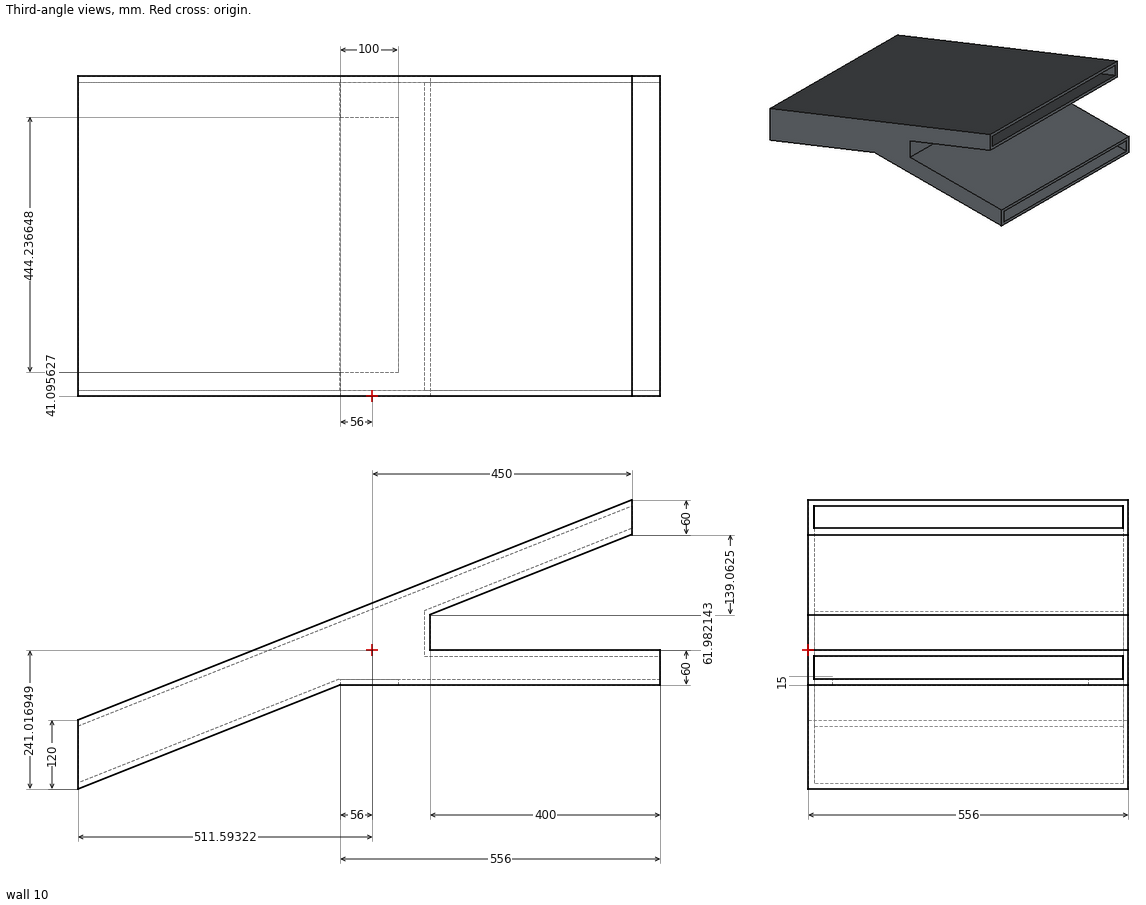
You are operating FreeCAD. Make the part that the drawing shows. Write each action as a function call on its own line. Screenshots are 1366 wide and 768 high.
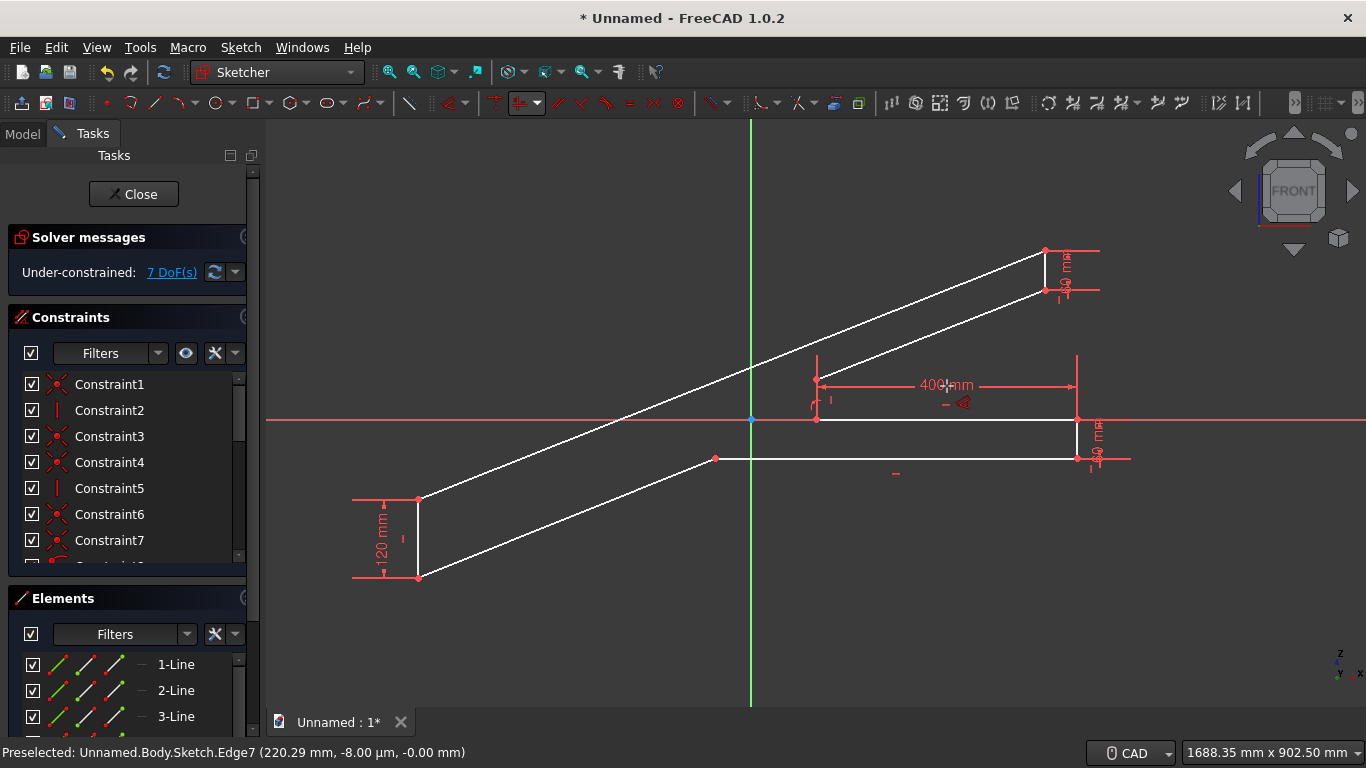
click(969, 459)
click(896, 493)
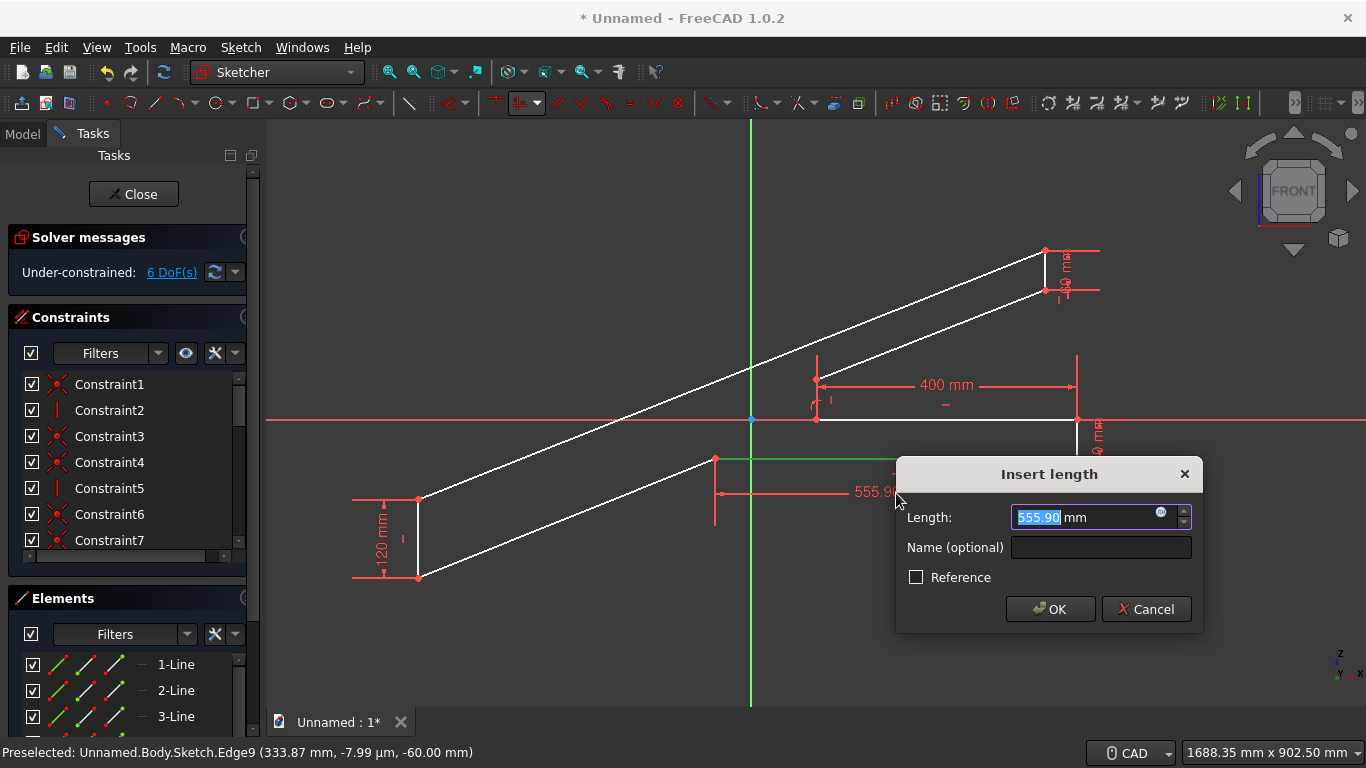
text(556)
key(Return)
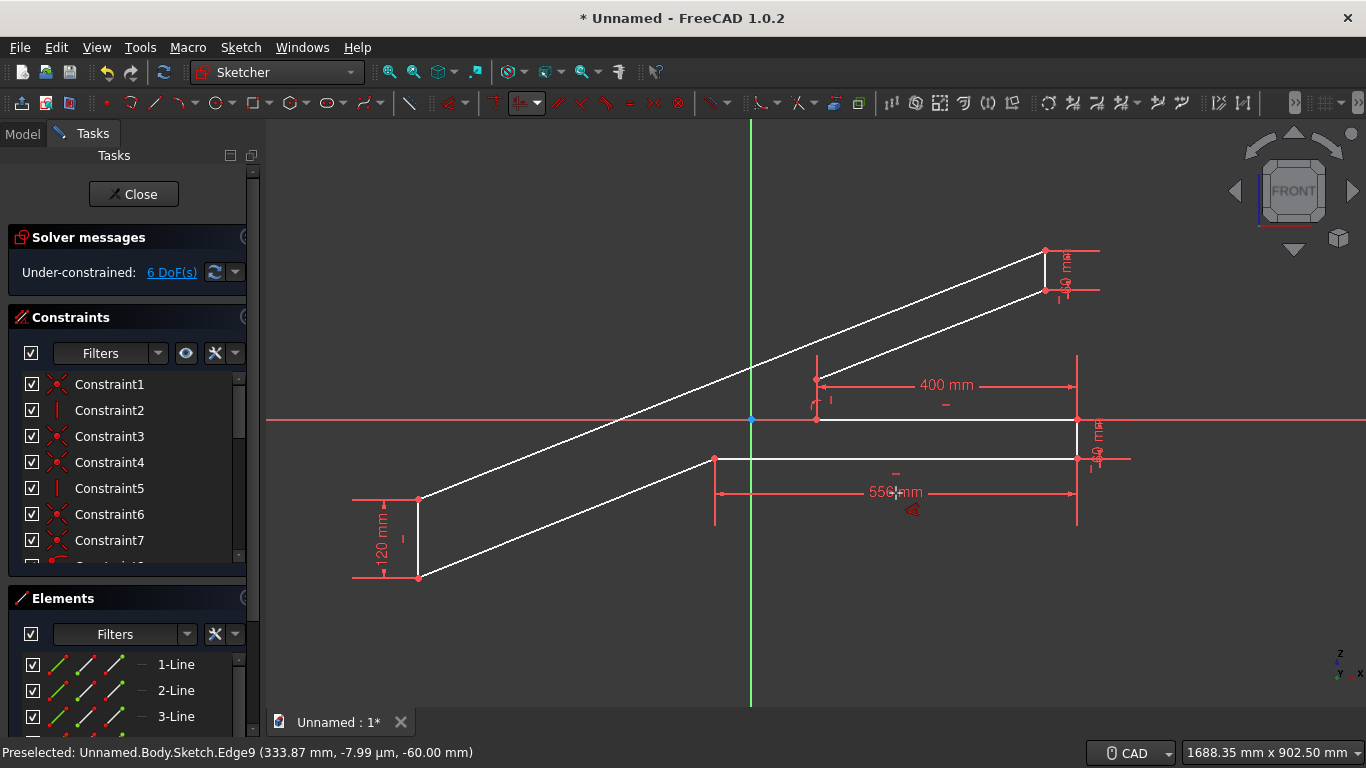
click(715, 459)
click(733, 493)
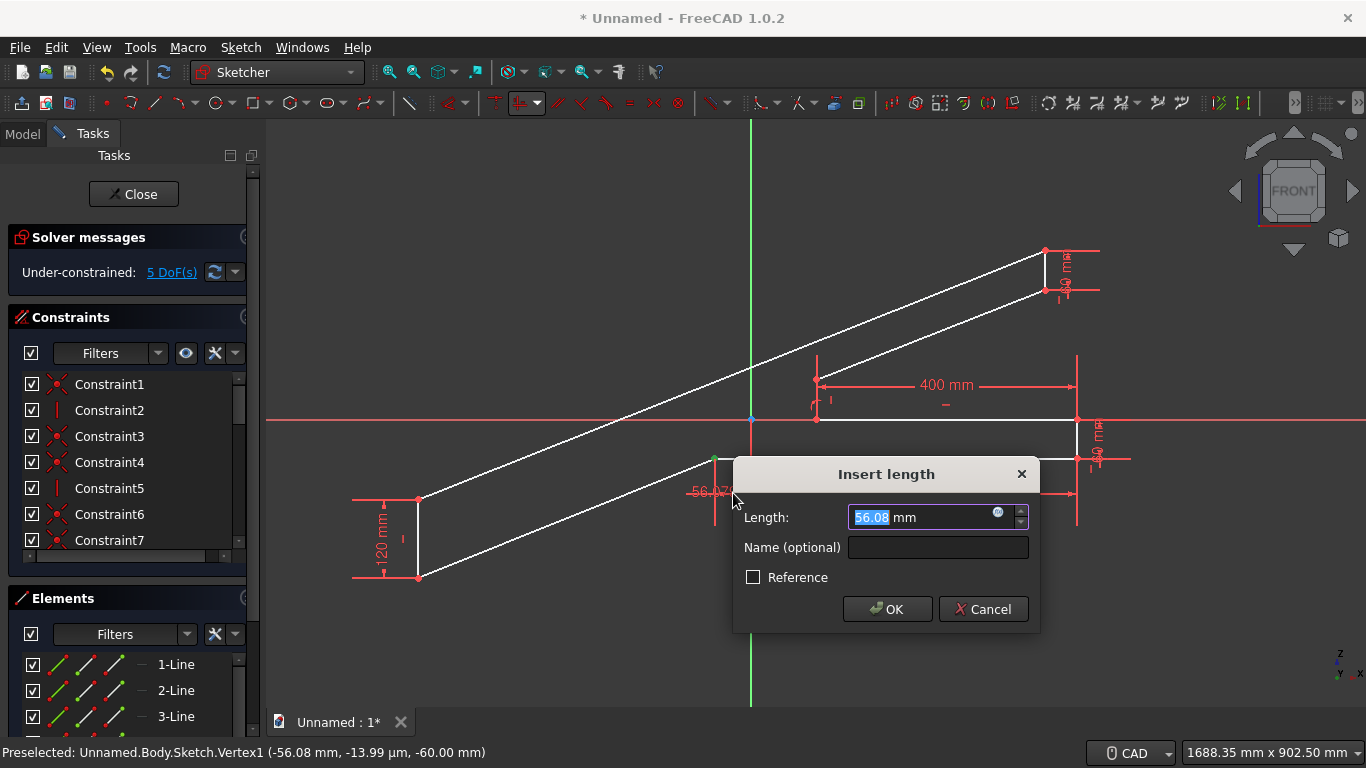
text(56)
key(Return)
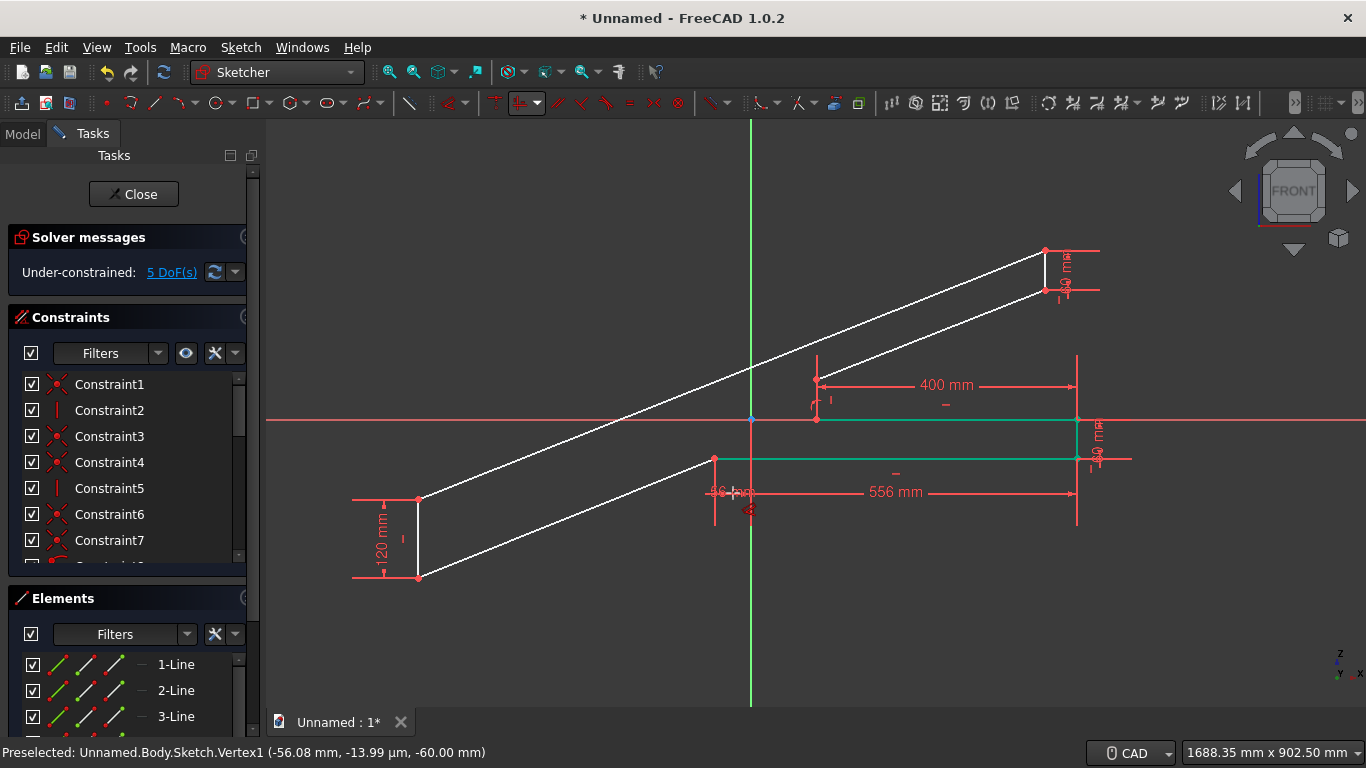
click(1045, 251)
click(898, 217)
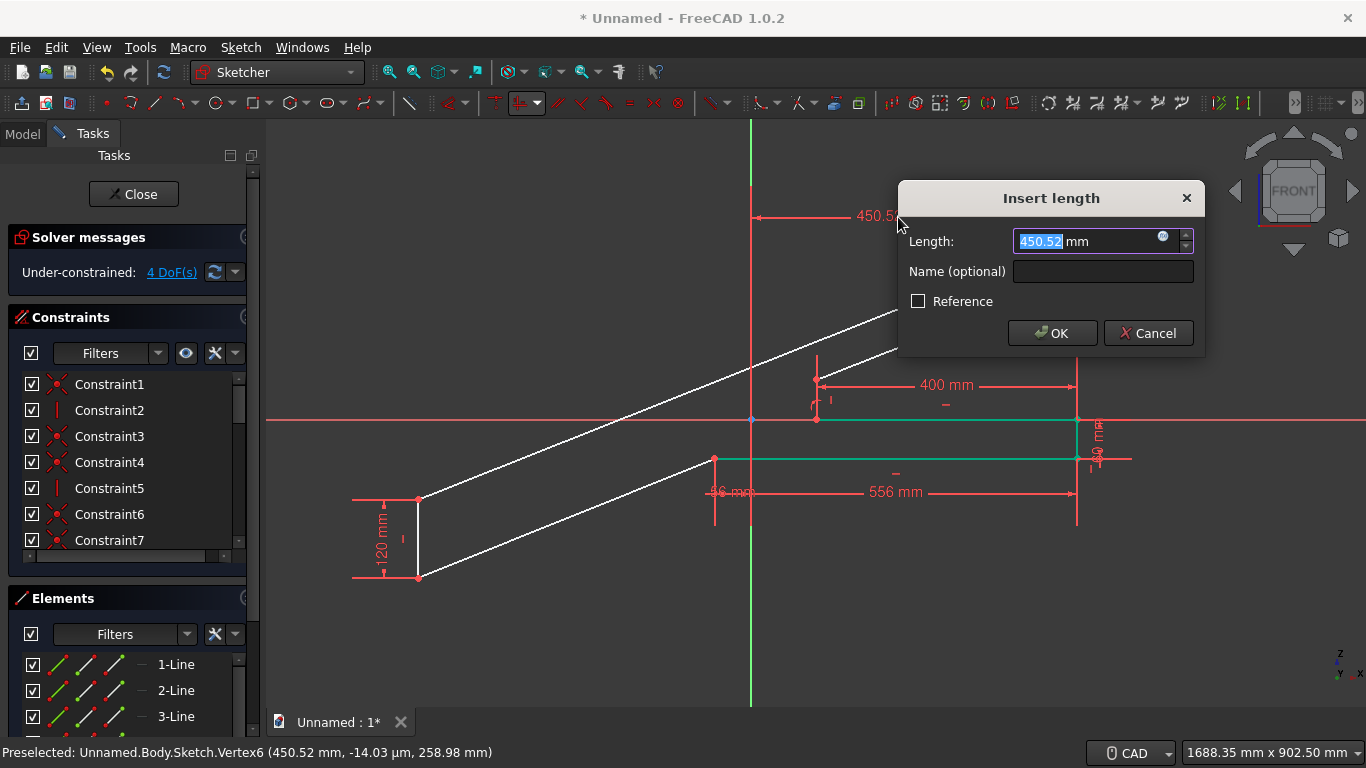
text(450)
key(Return)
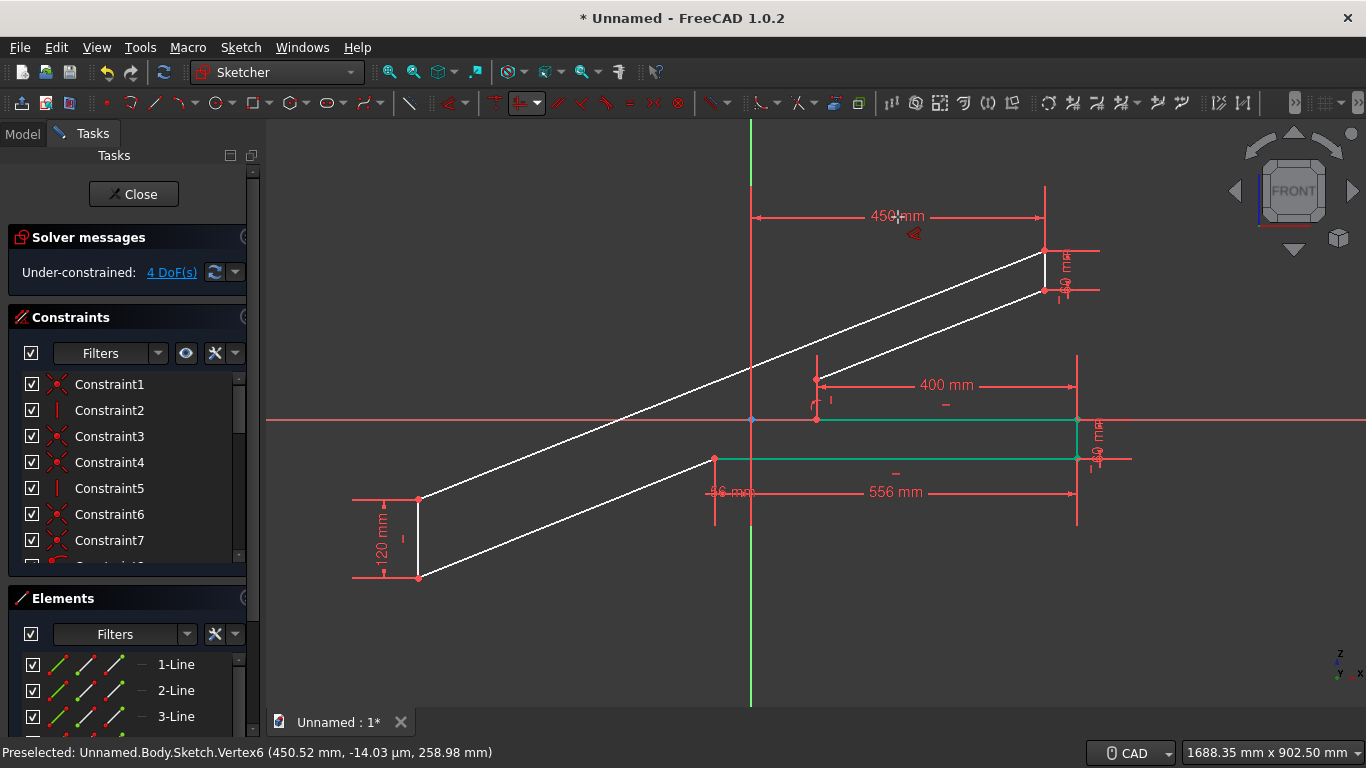
click(817, 392)
click(851, 400)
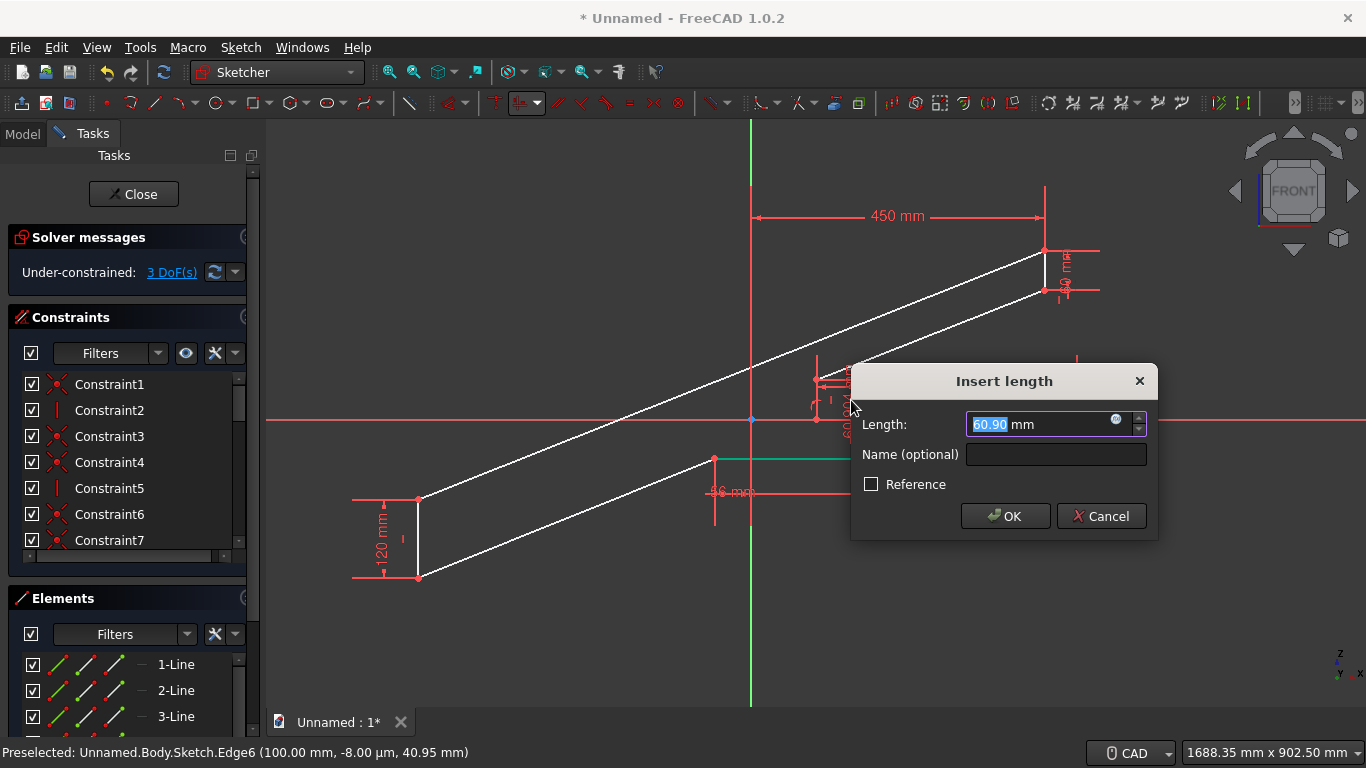
text(61.982143)
key(Return)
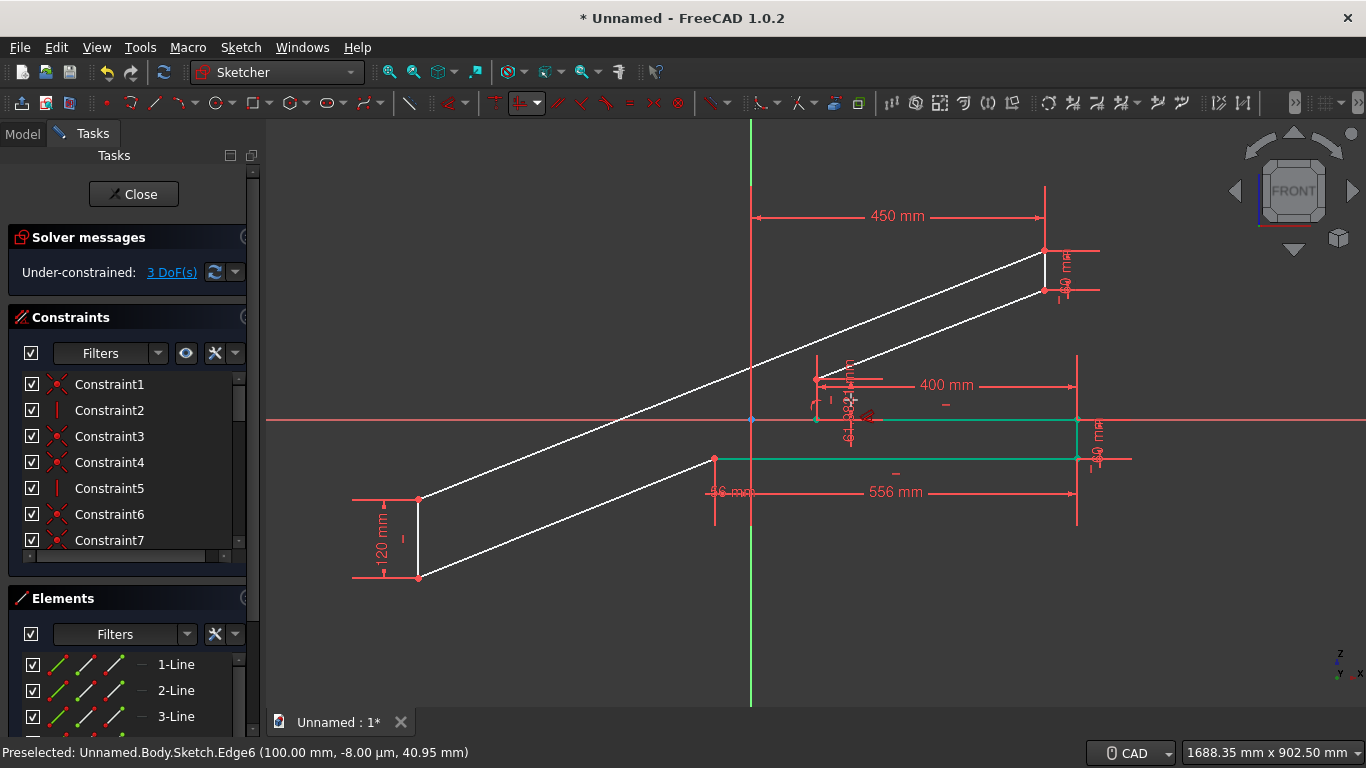
click(976, 317)
click(1079, 335)